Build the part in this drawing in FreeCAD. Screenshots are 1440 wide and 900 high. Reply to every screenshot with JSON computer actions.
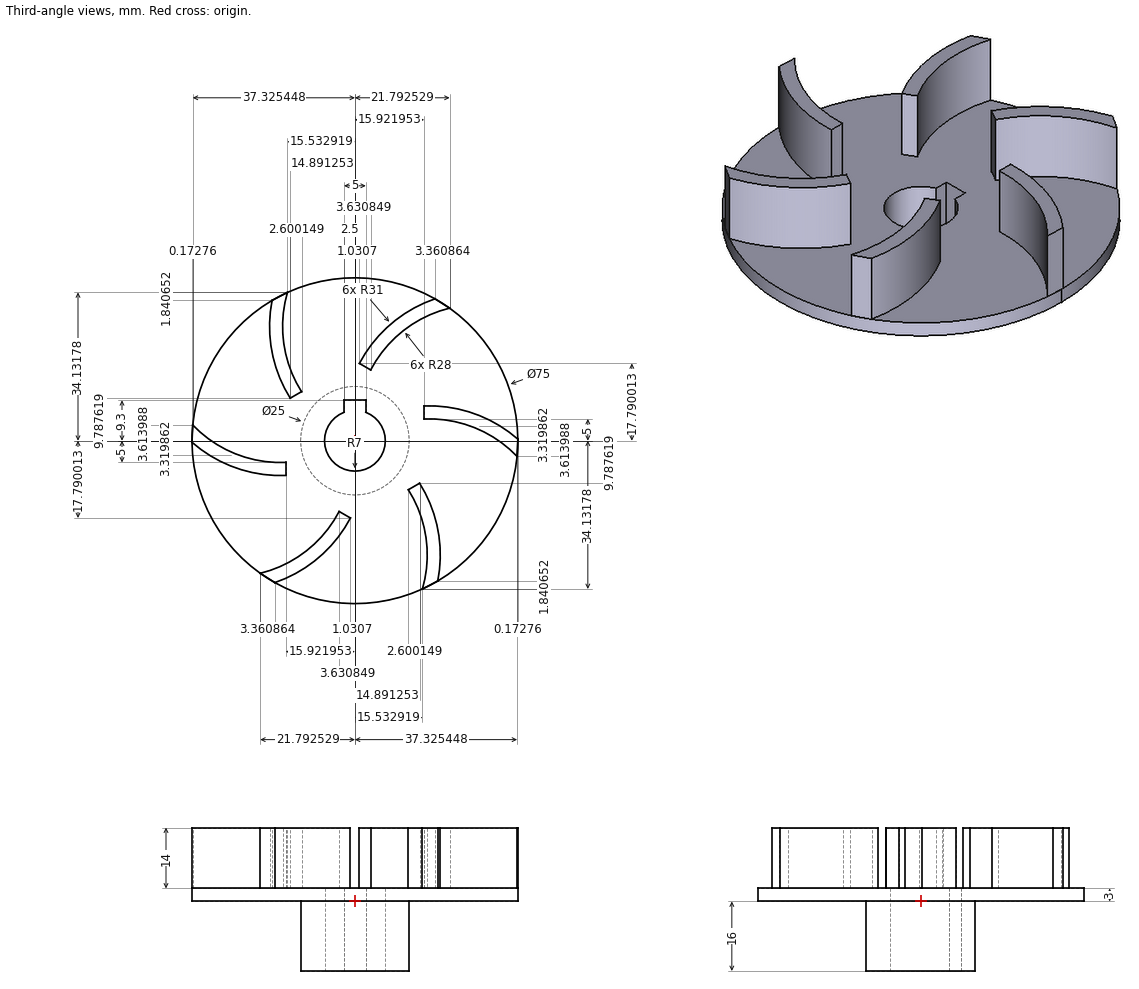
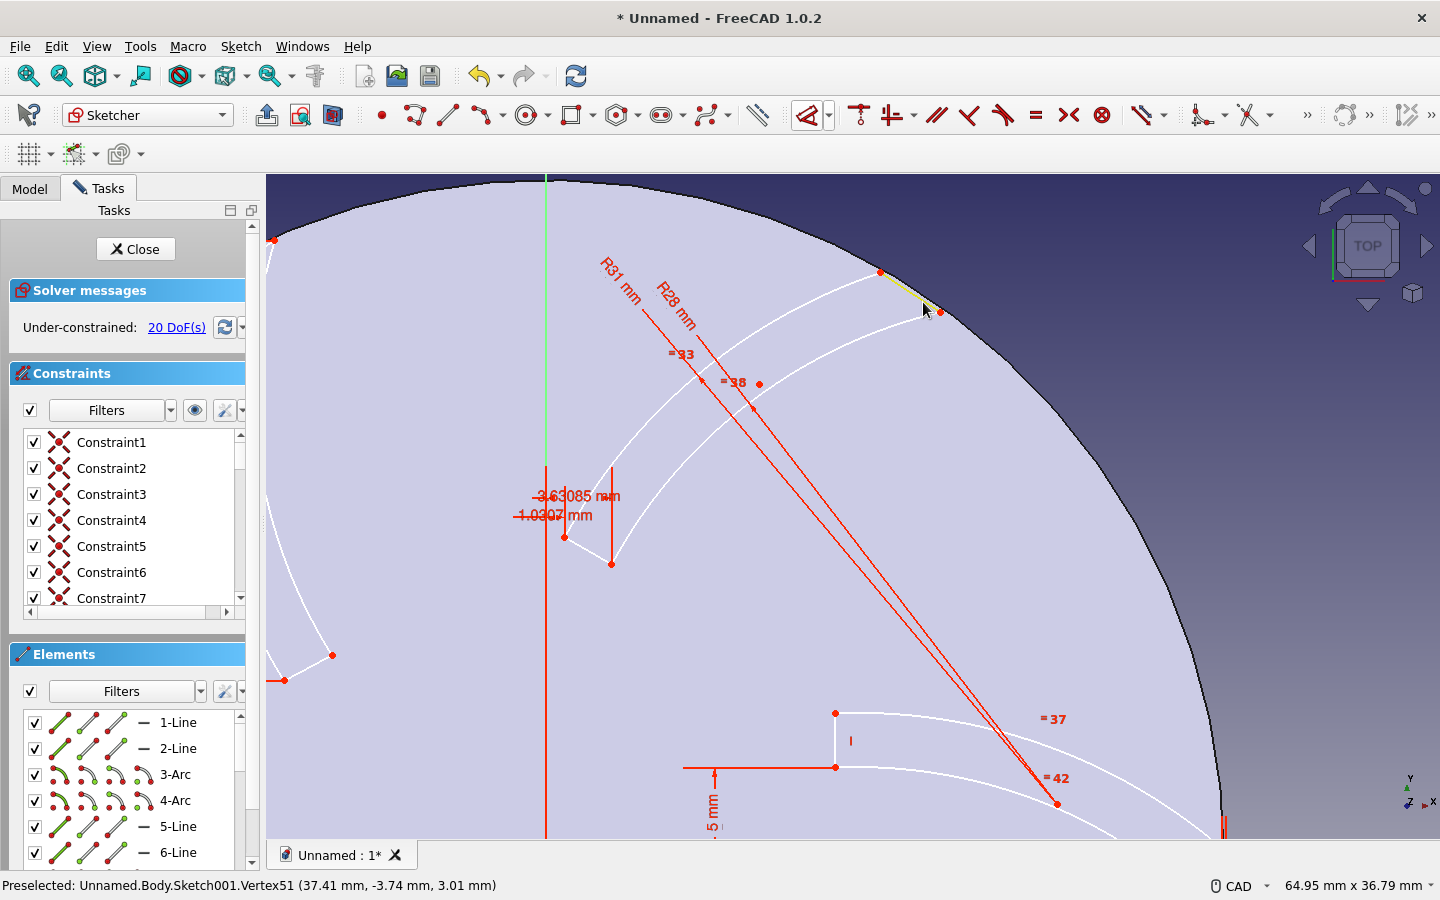
{"action": "left_click", "coordinate": [922, 300]}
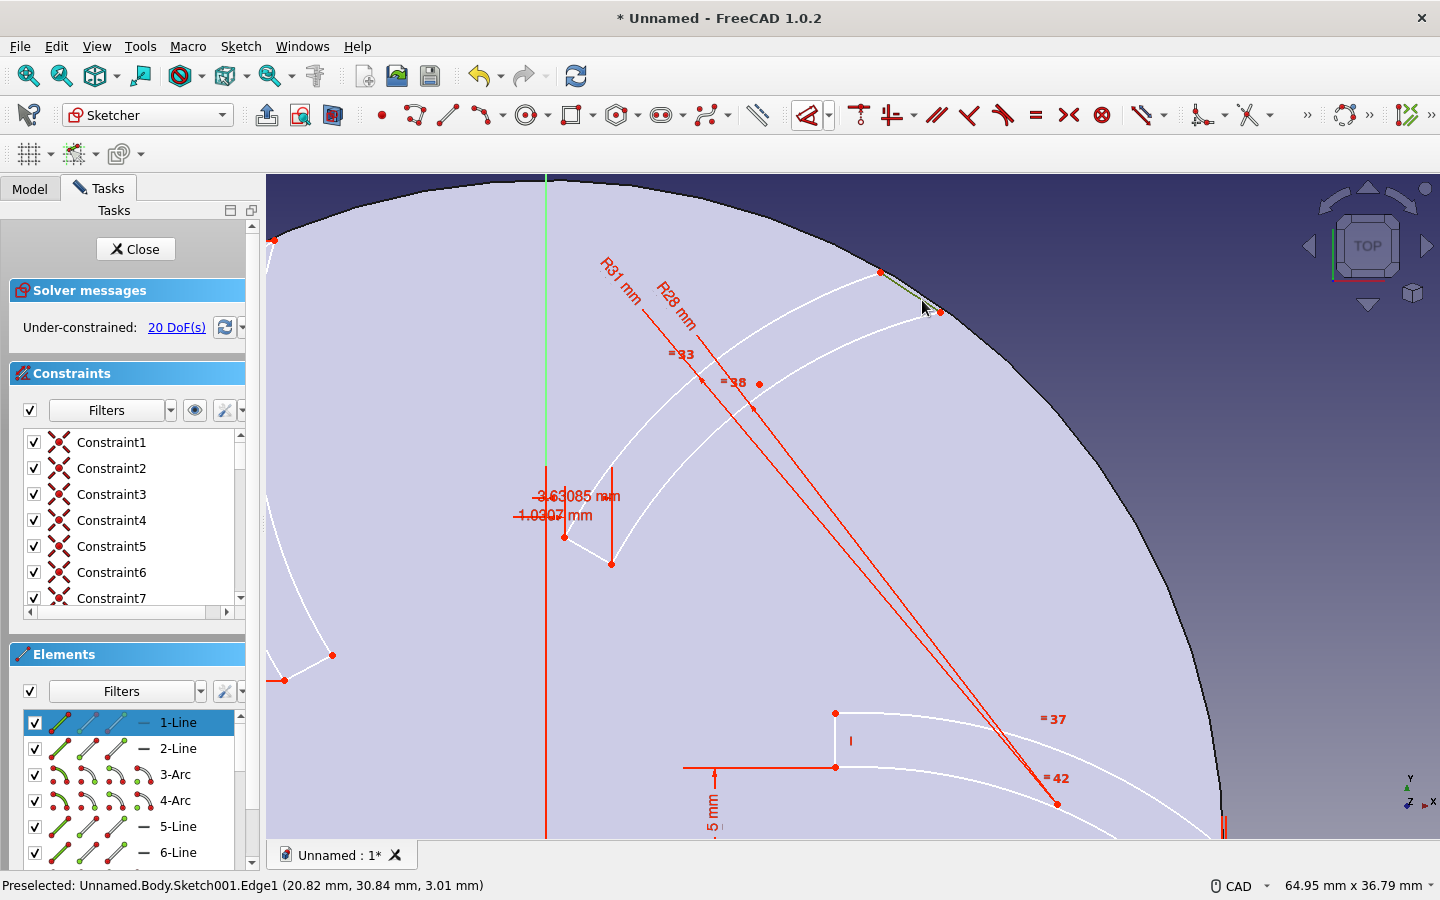
{"action": "key", "text": "l"}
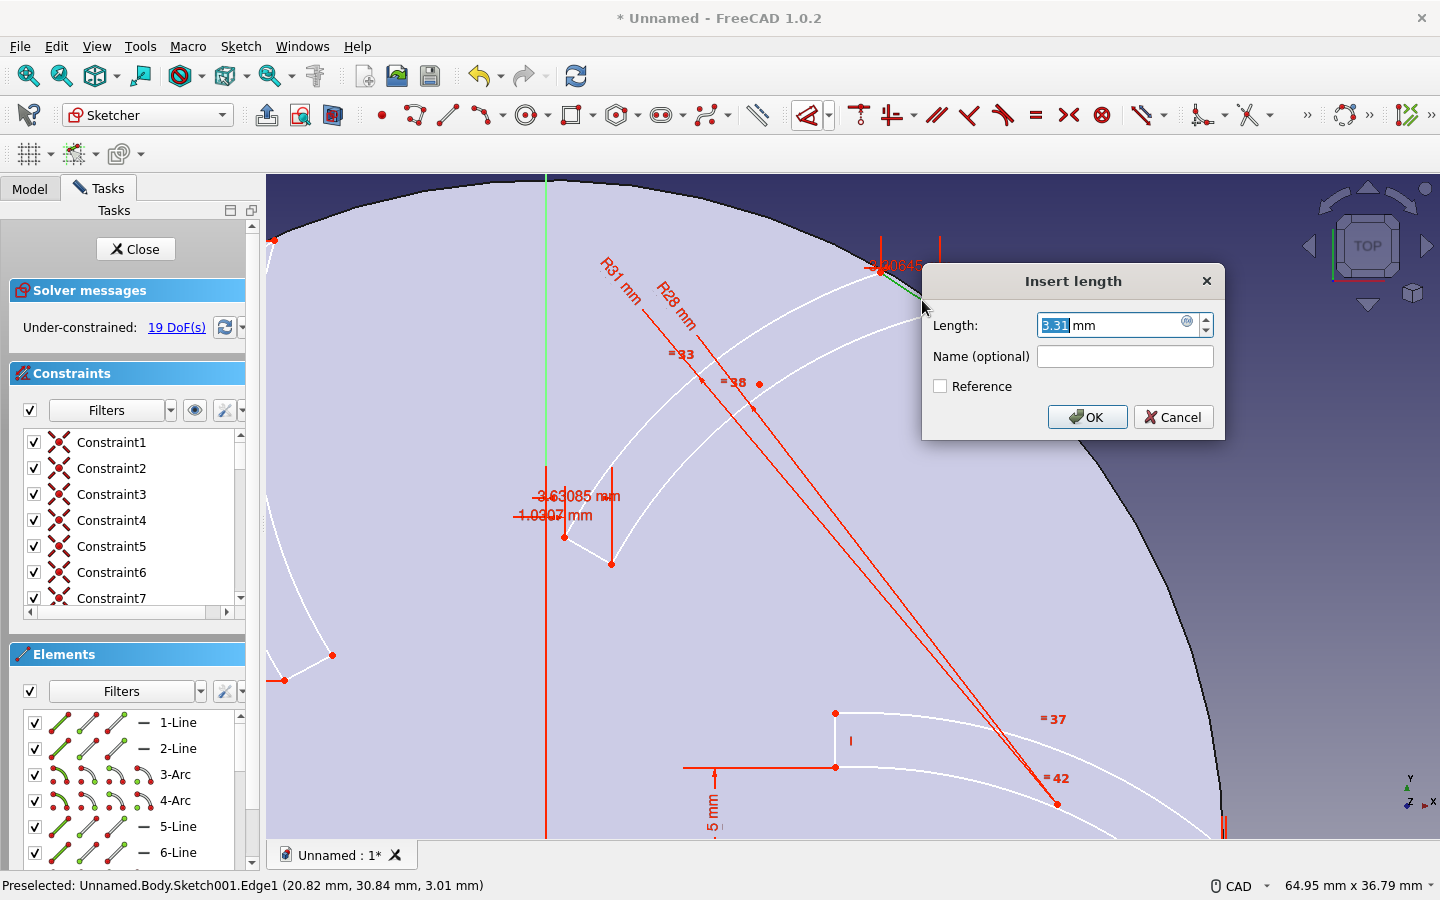
{"action": "type", "text": "3.360864"}
{"action": "key", "text": "Return"}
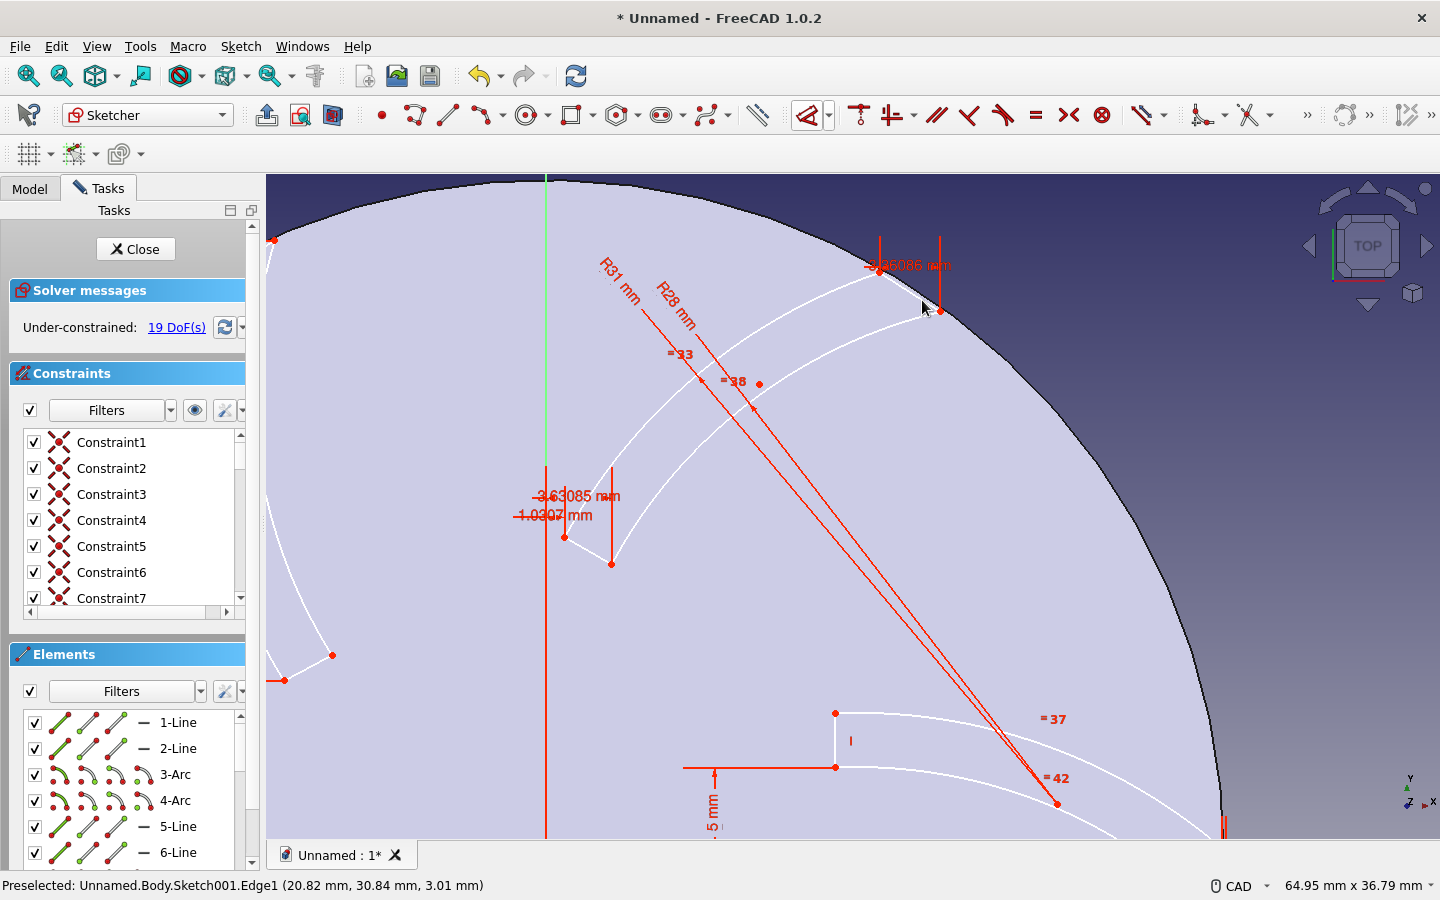
{"action": "scroll", "coordinate": [923, 302], "scroll_direction": "down", "scroll_amount": 5}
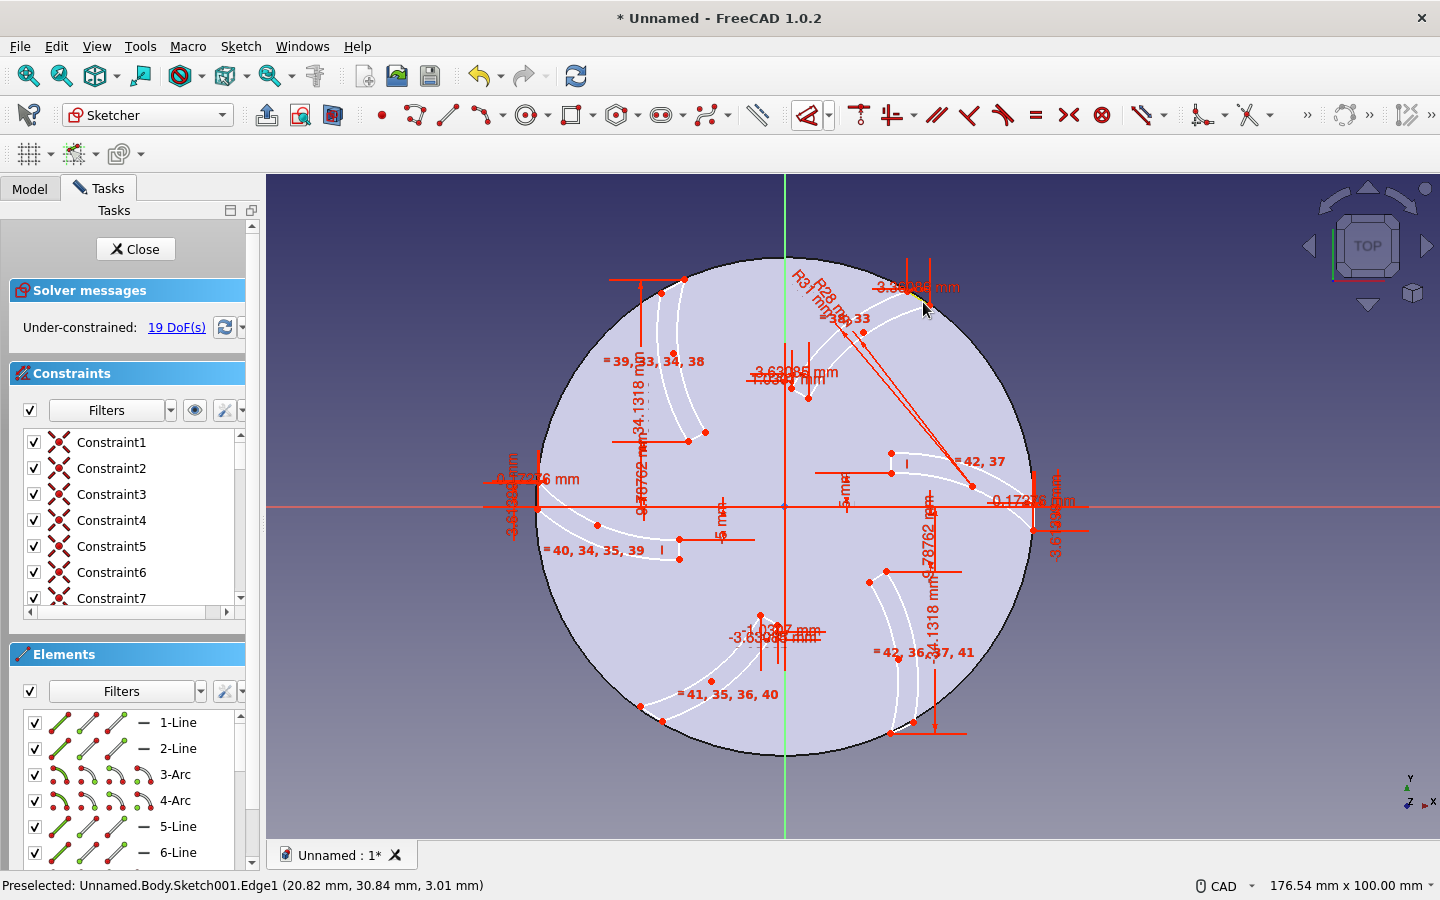
{"action": "scroll", "coordinate": [678, 284], "scroll_direction": "up", "scroll_amount": 6}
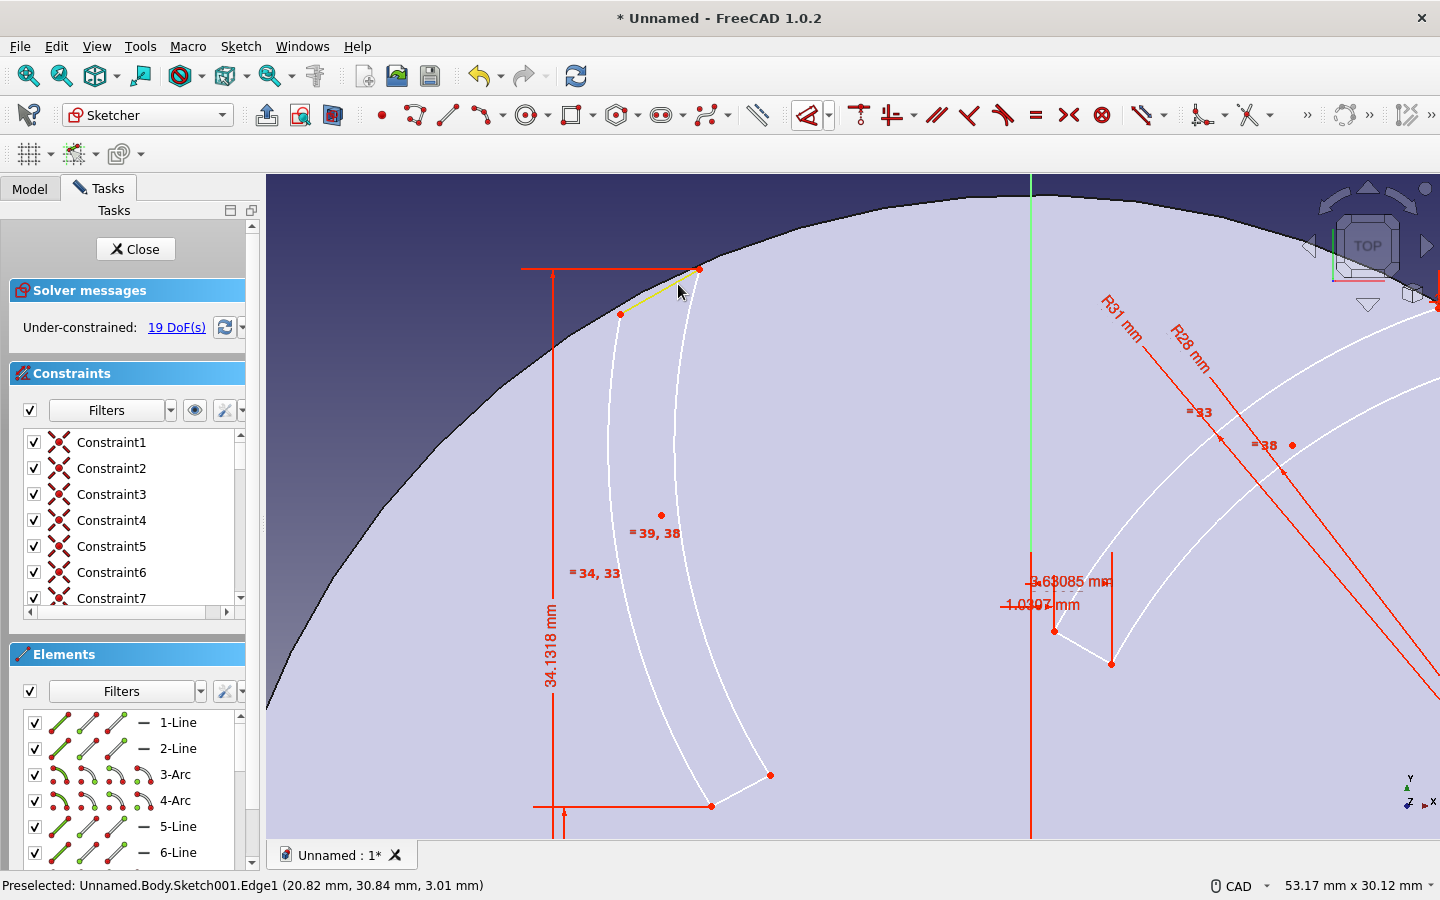
{"action": "left_click", "coordinate": [676, 283]}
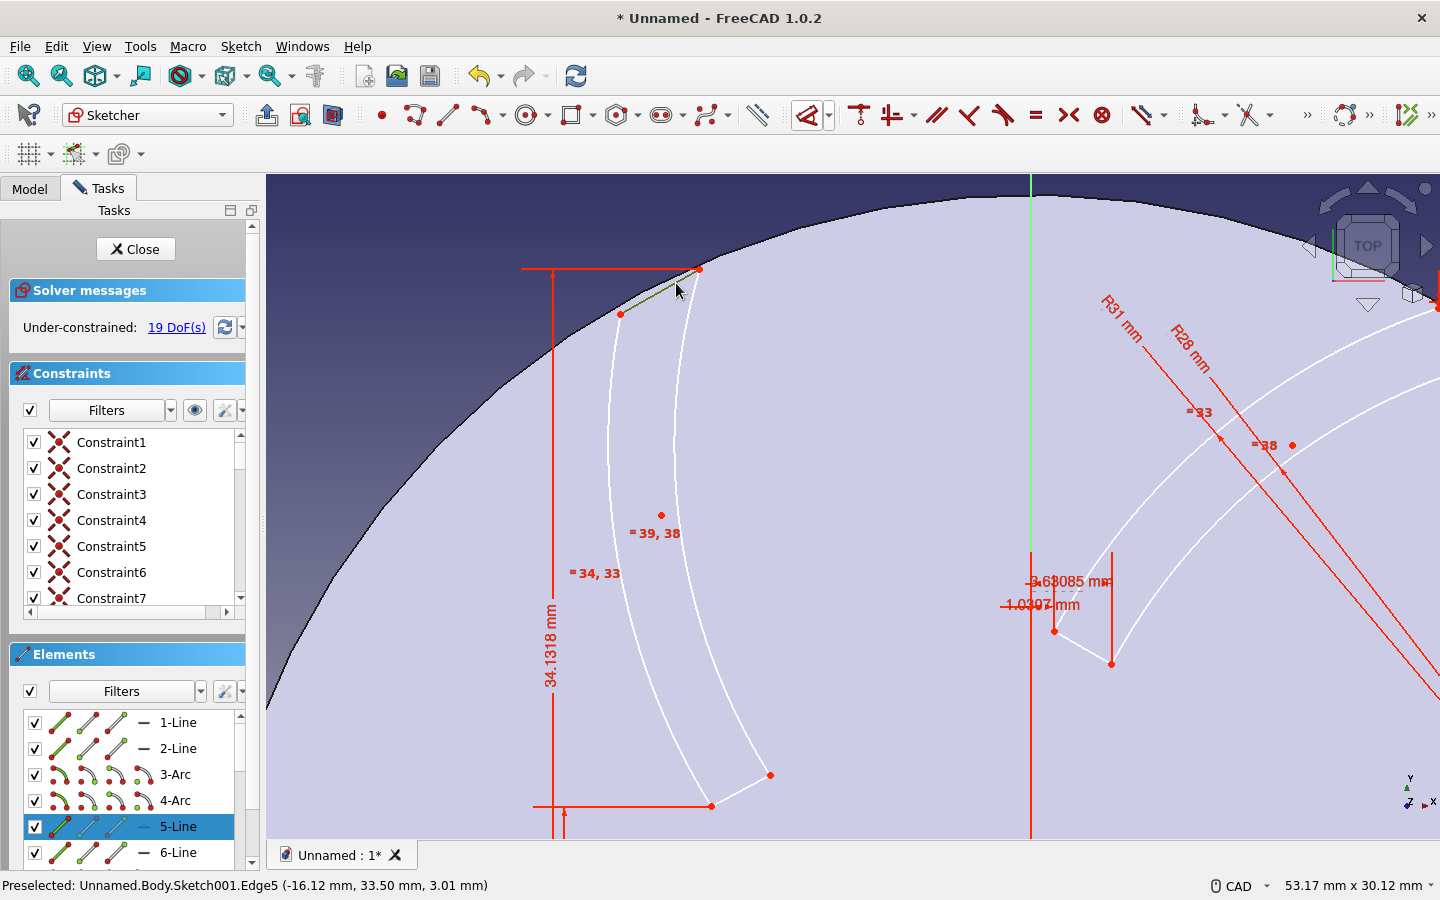
{"action": "key", "text": "i"}